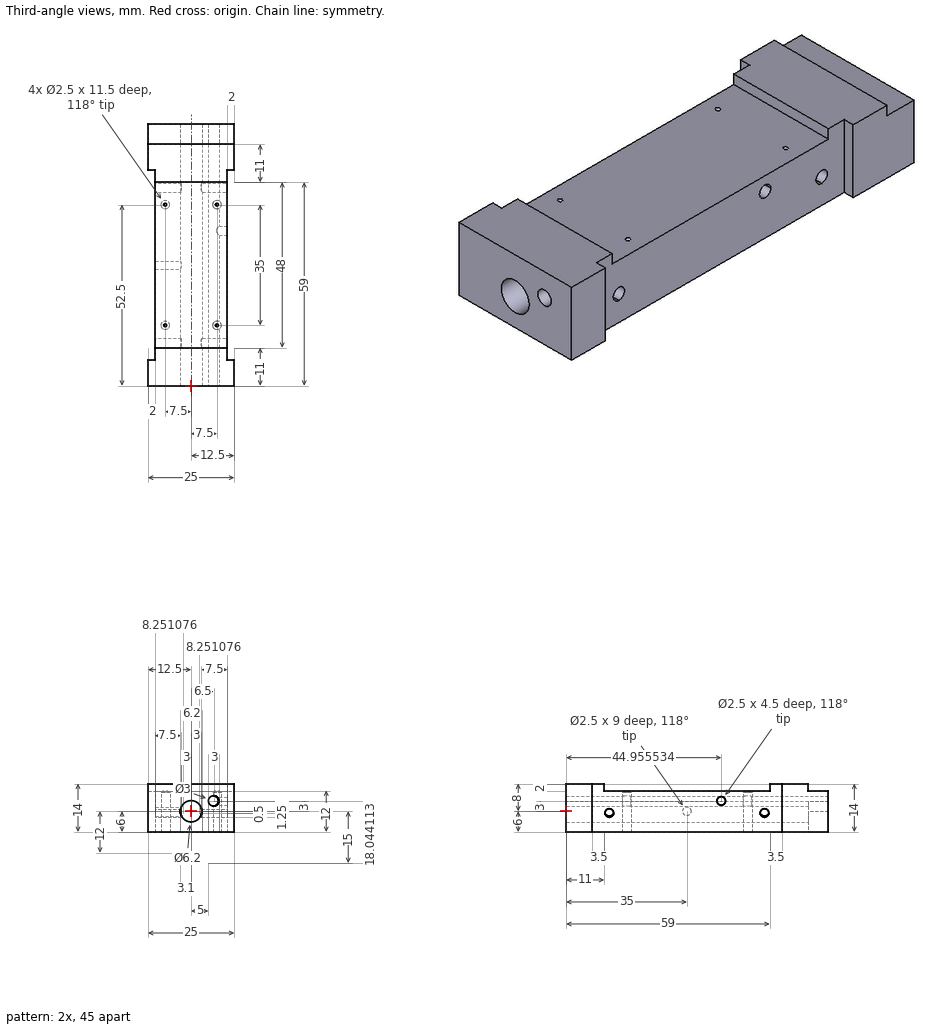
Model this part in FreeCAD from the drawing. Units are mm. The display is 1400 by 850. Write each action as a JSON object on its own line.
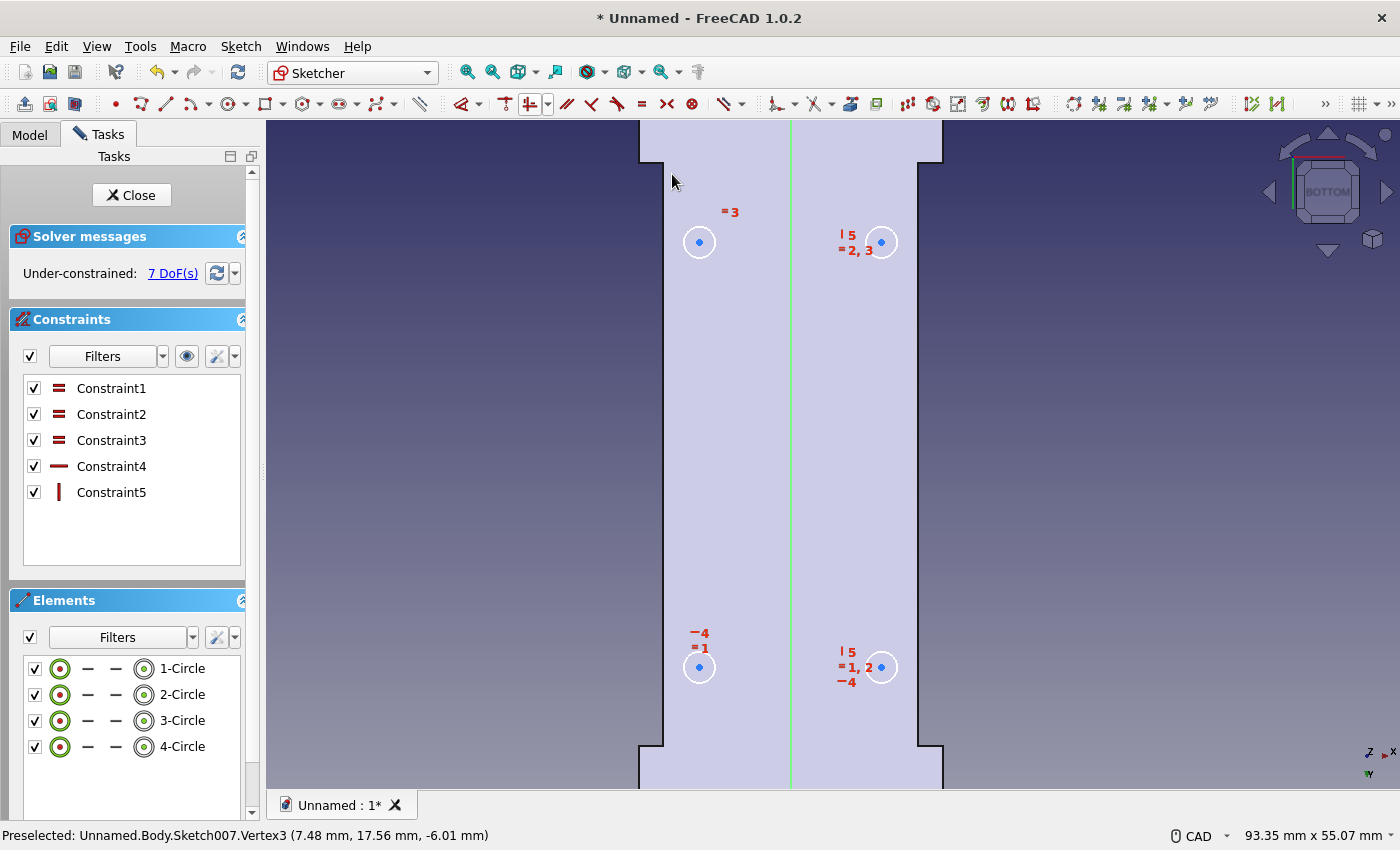
{"action": "left_click", "coordinate": [699, 667]}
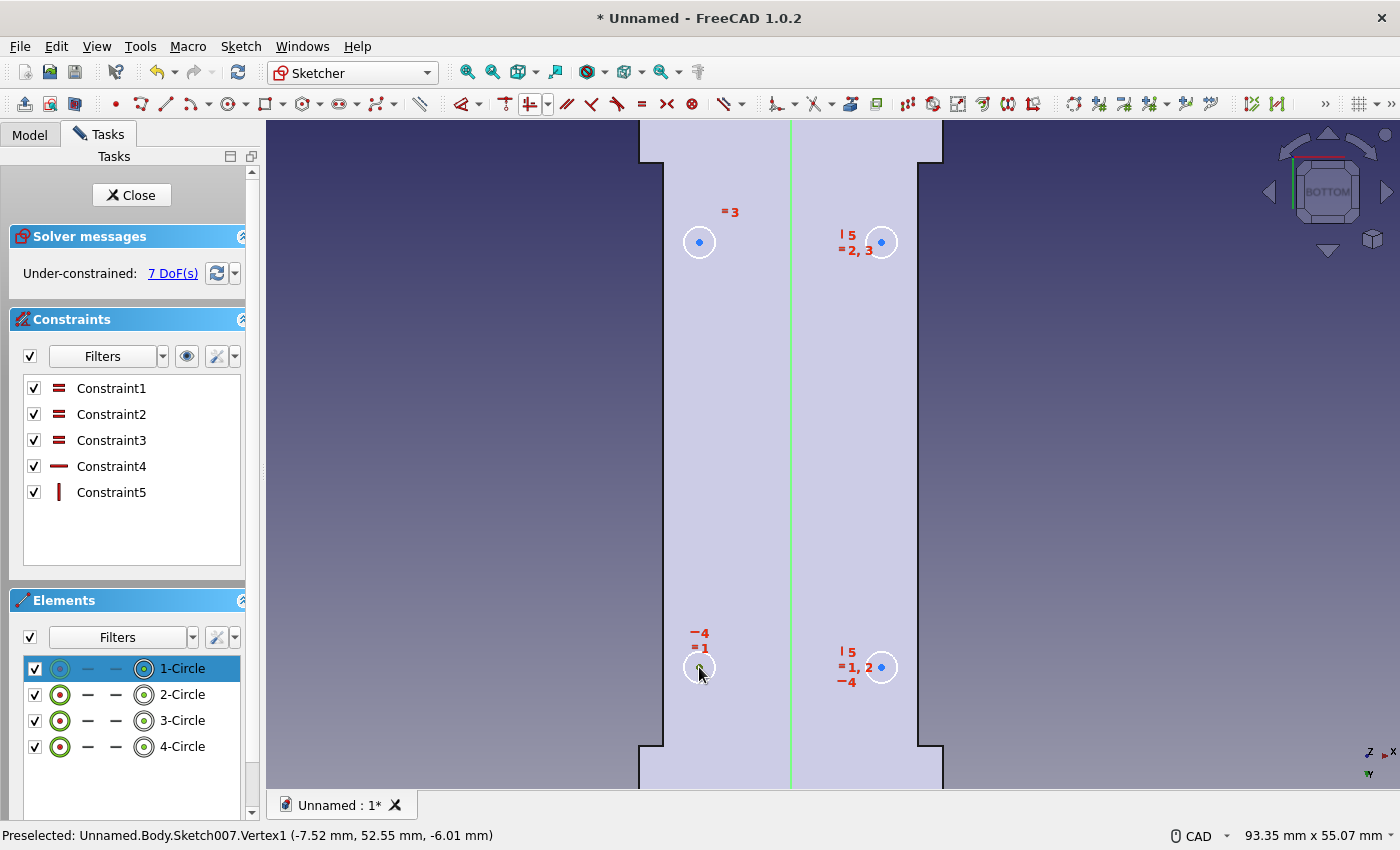
{"action": "left_click", "coordinate": [700, 242]}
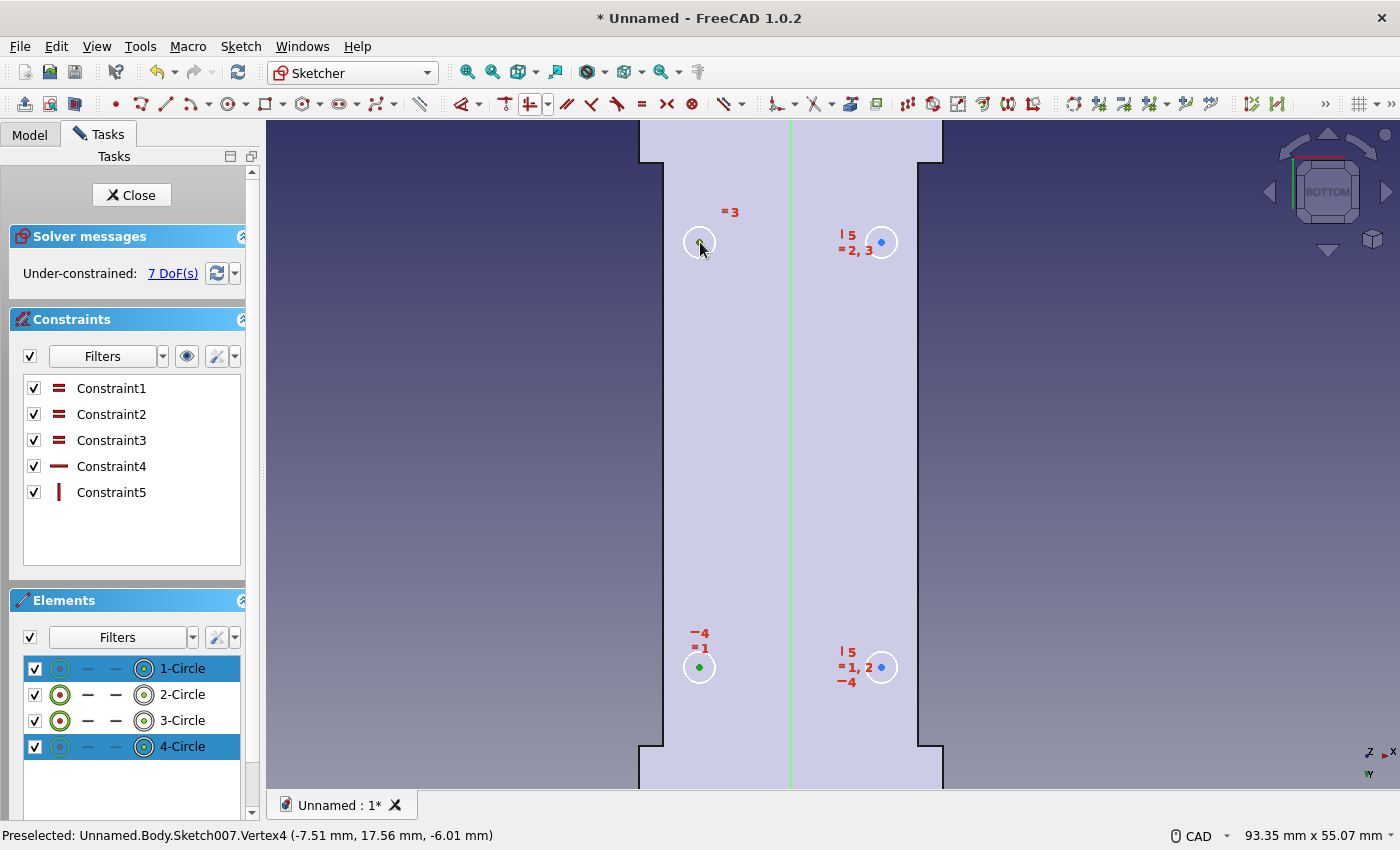
{"action": "left_click", "coordinate": [548, 104]}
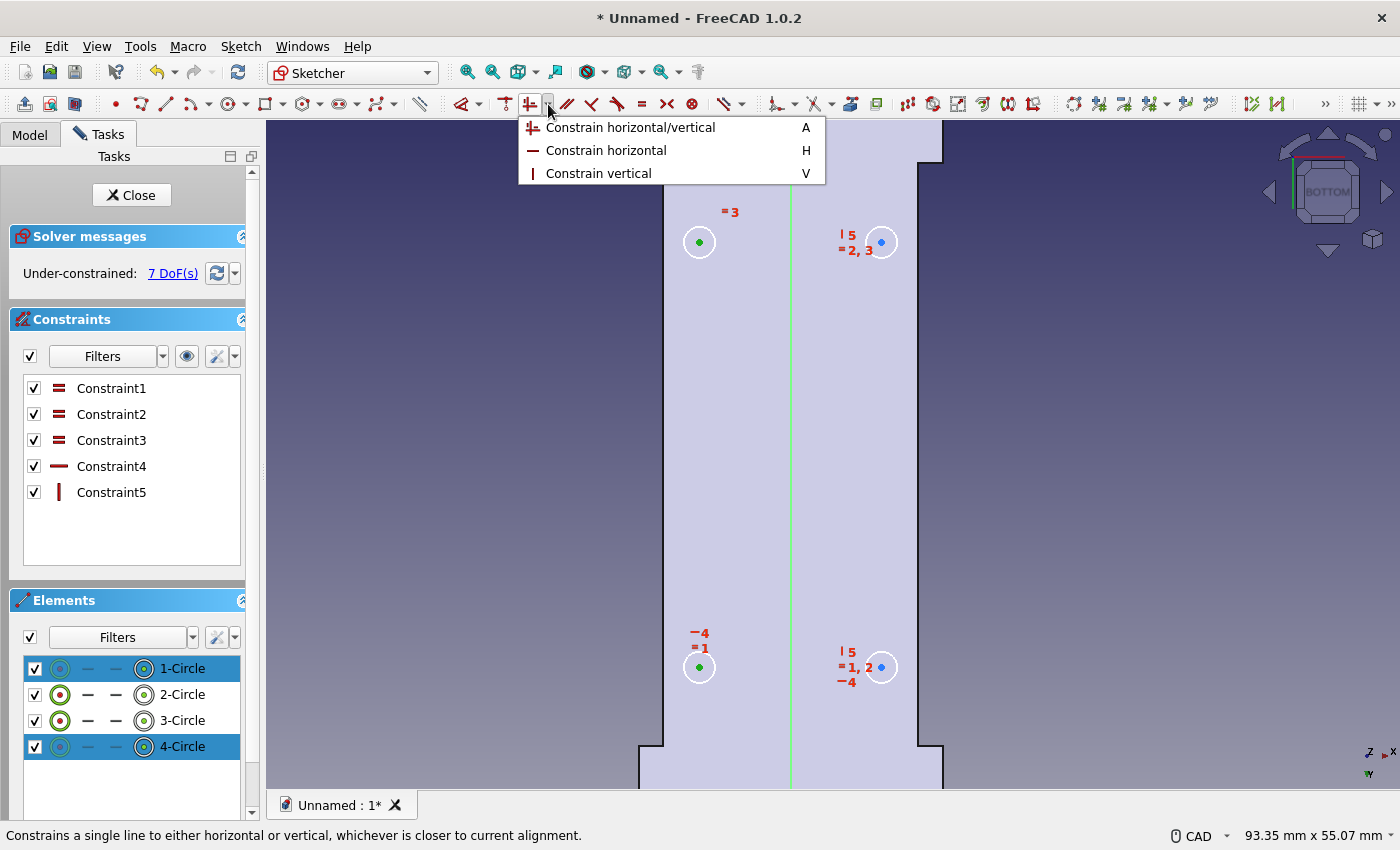
{"action": "left_click", "coordinate": [672, 174]}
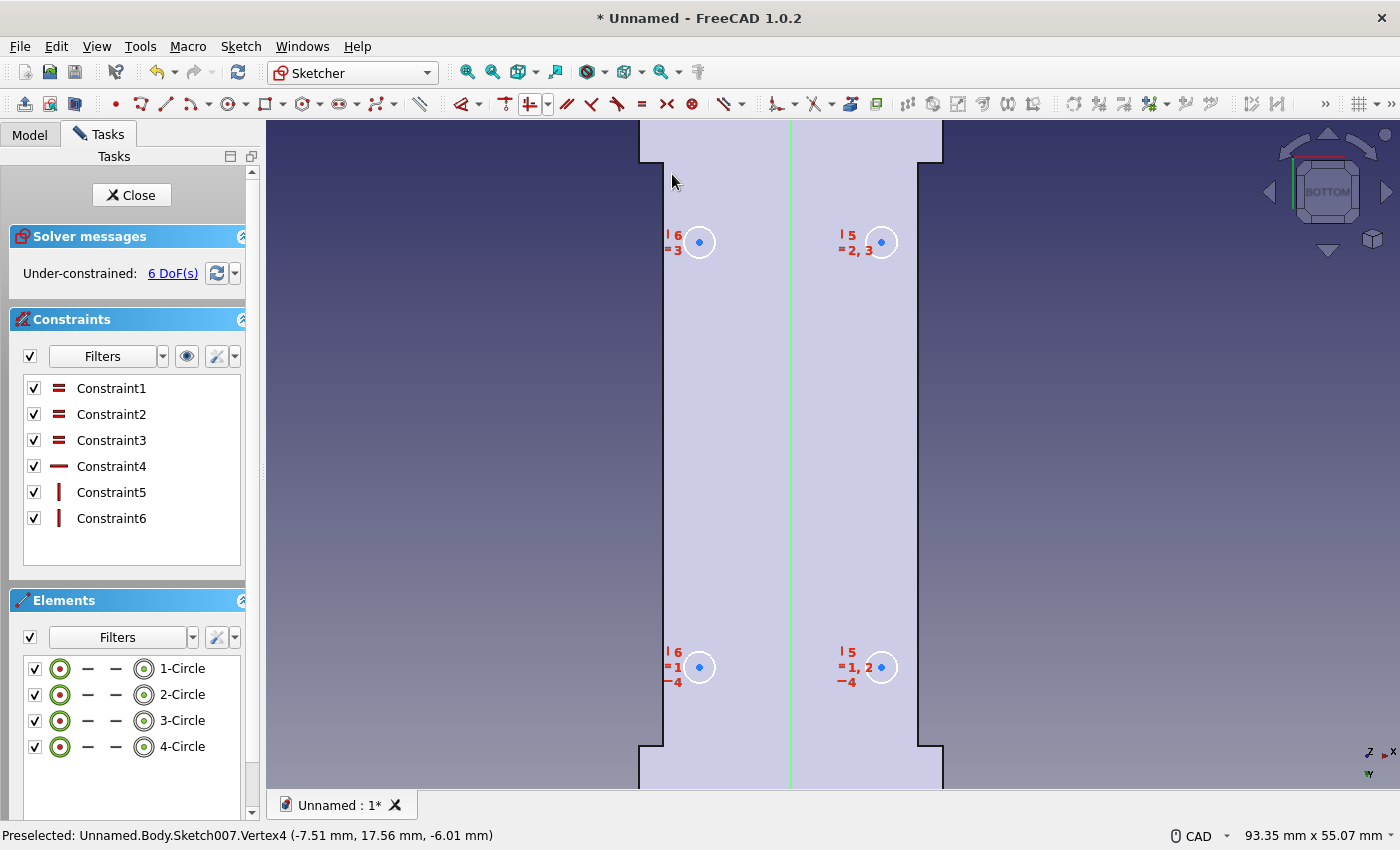
{"action": "left_click", "coordinate": [882, 242]}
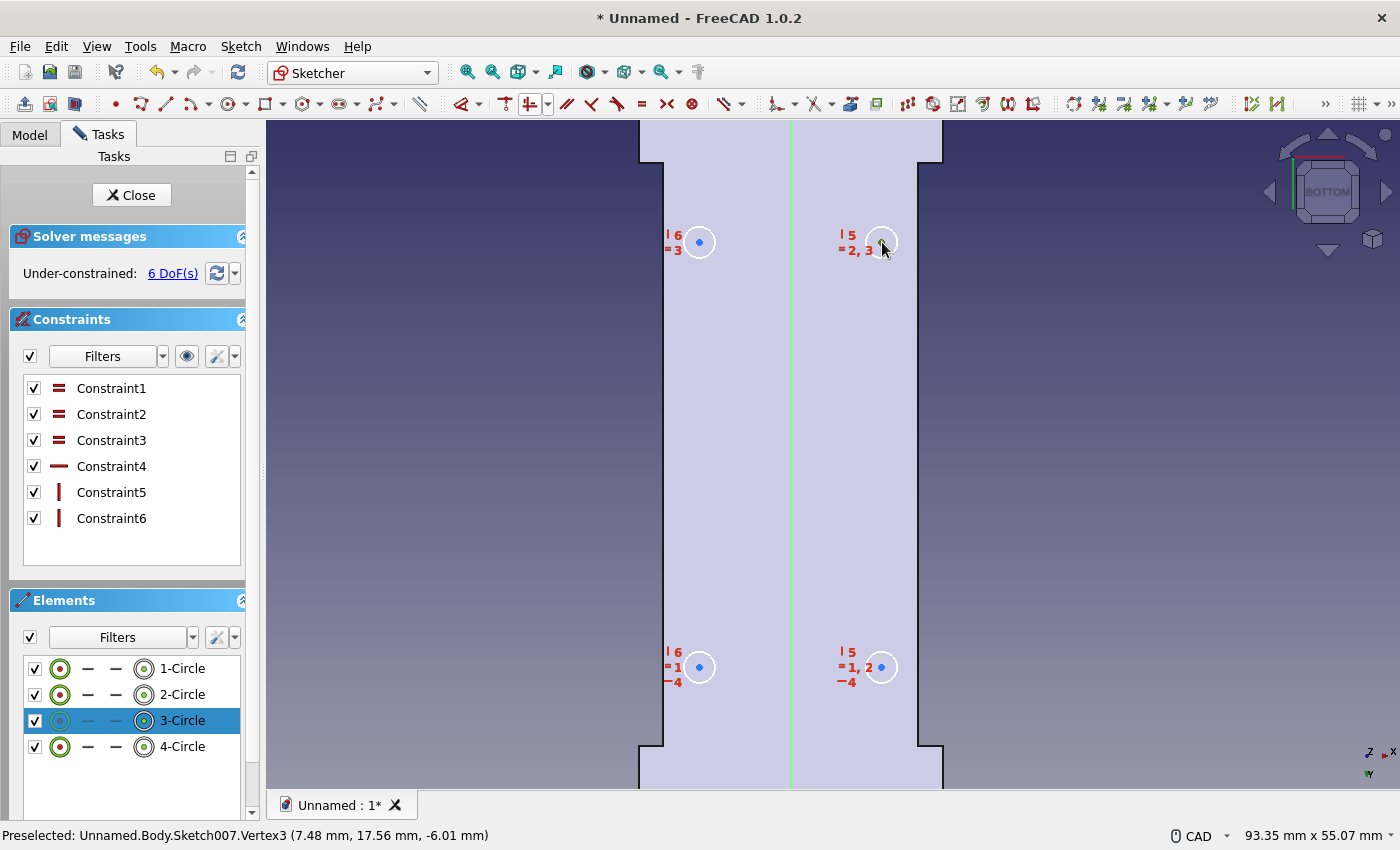
{"action": "left_click", "coordinate": [699, 242]}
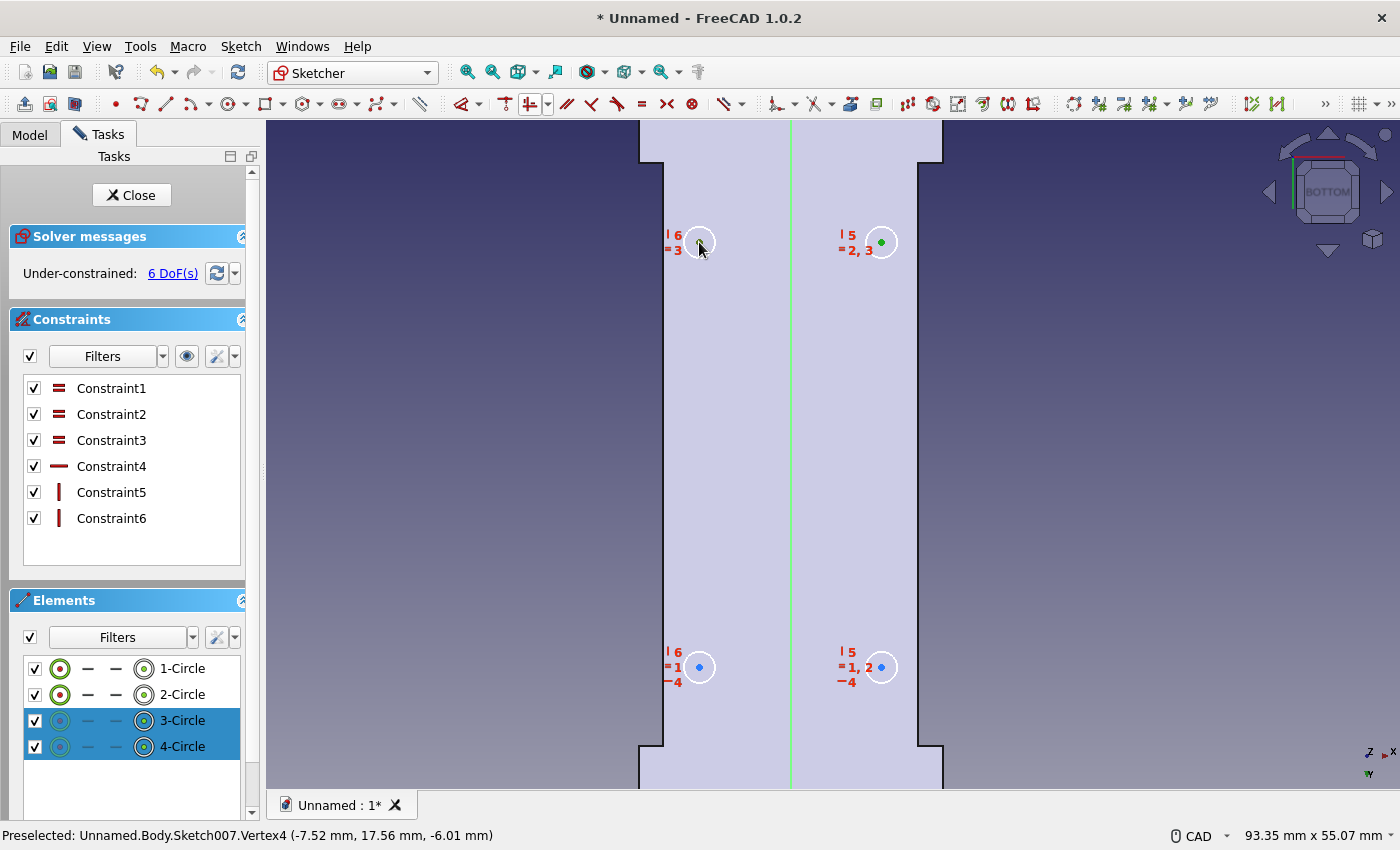
{"action": "left_click", "coordinate": [548, 104]}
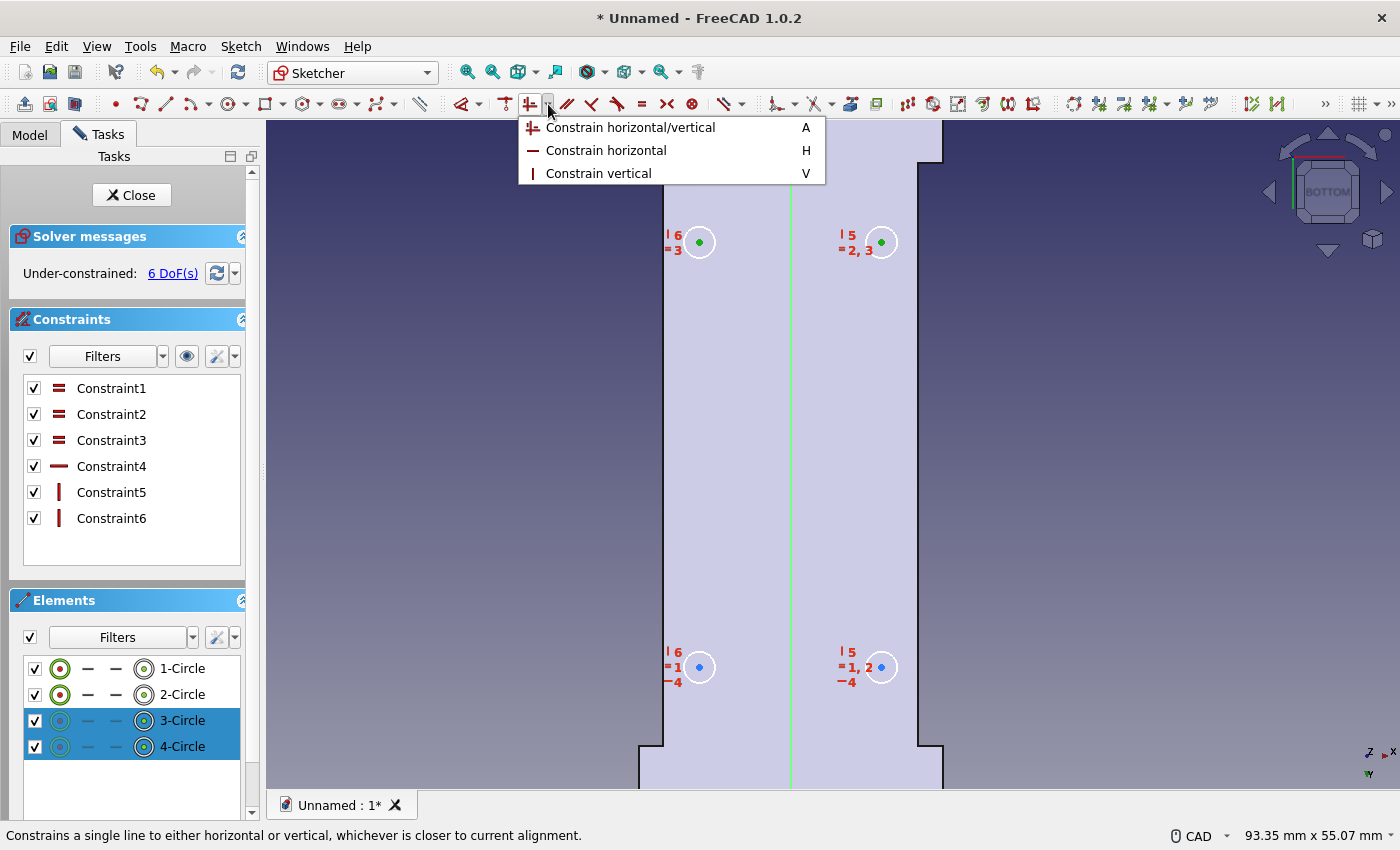
{"action": "left_click", "coordinate": [672, 150]}